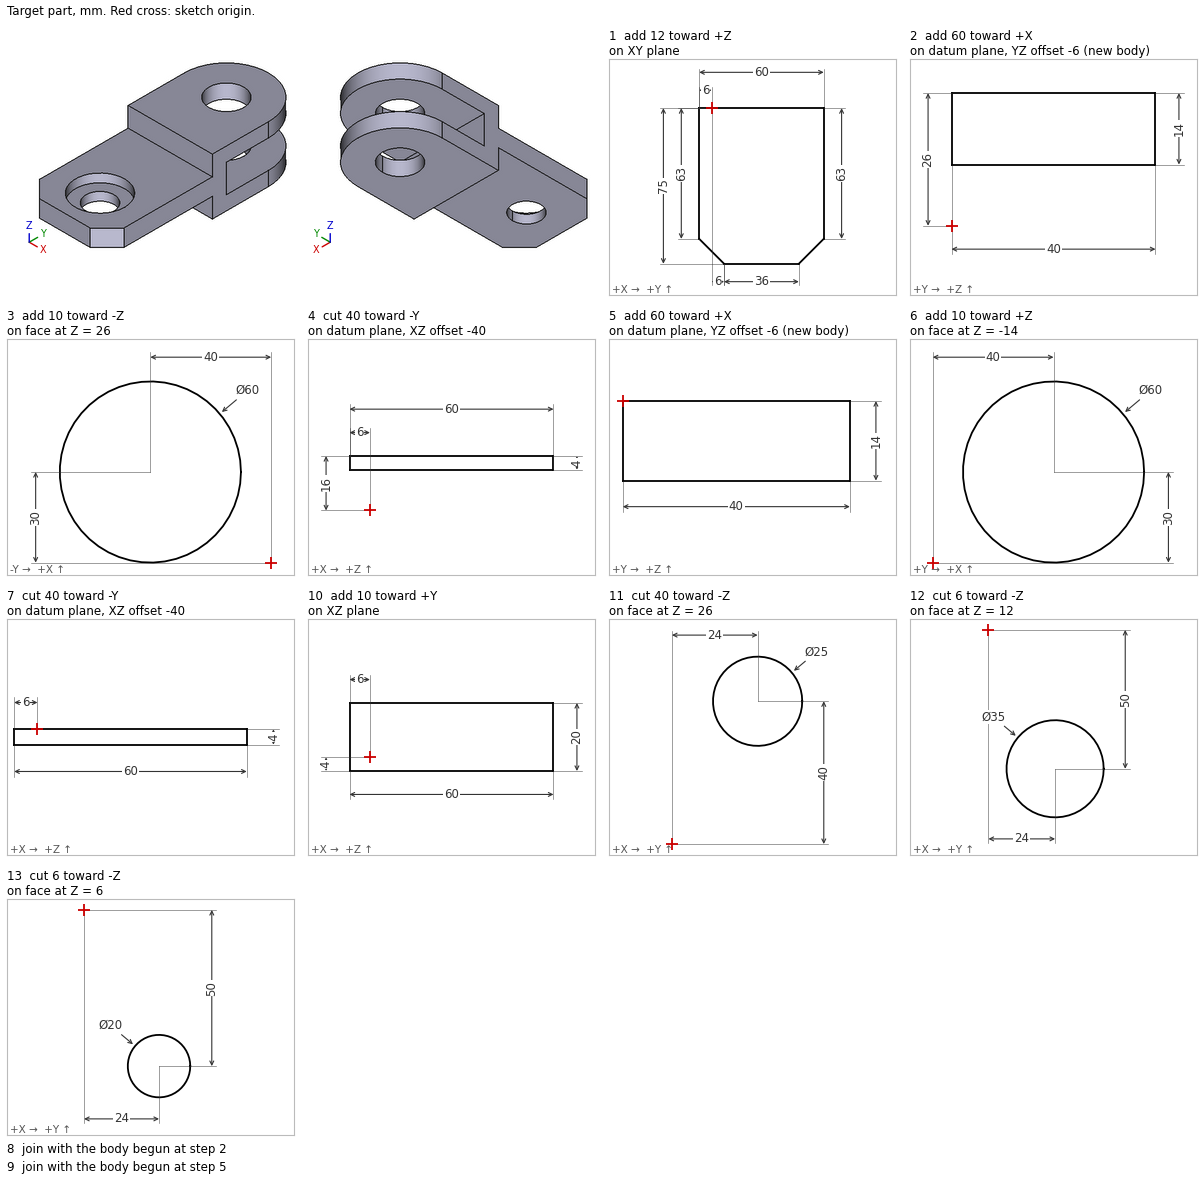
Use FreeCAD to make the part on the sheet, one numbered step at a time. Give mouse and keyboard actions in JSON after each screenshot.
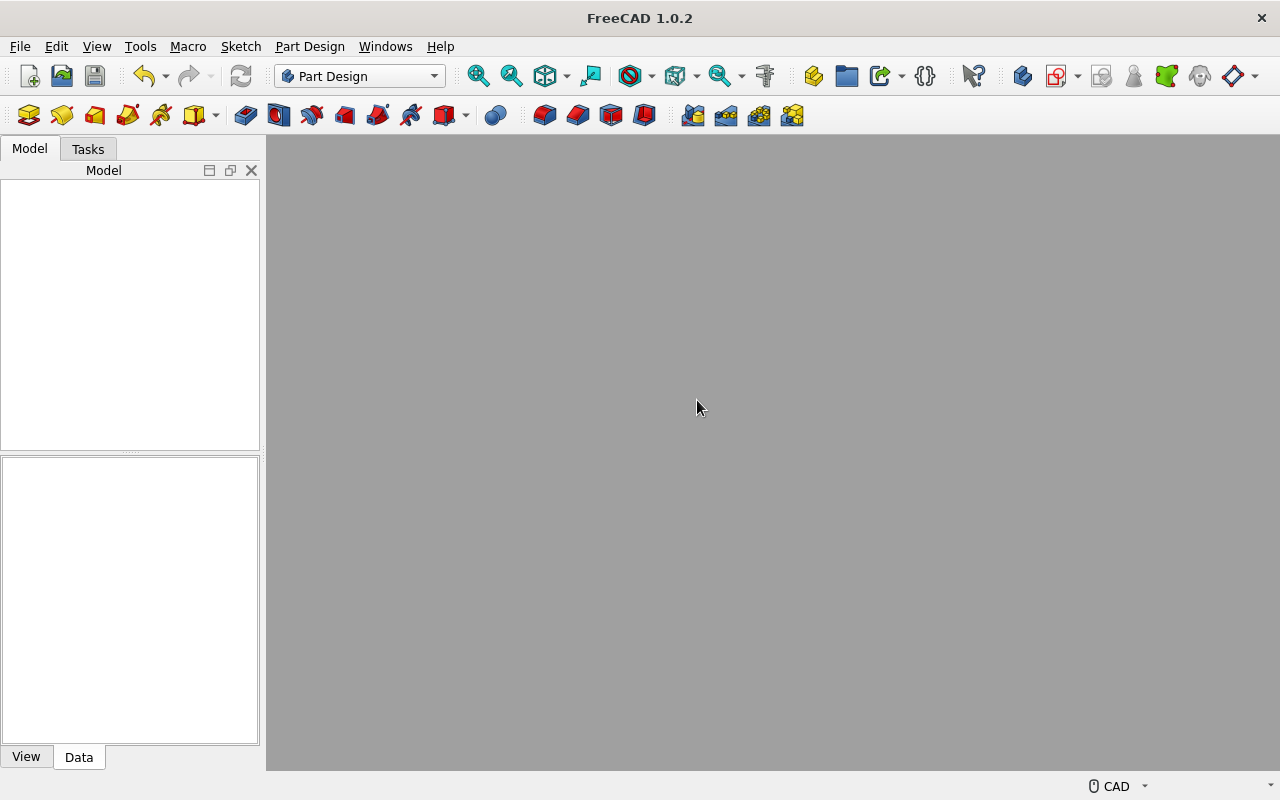
{"action": "left_click", "coordinate": [29, 76]}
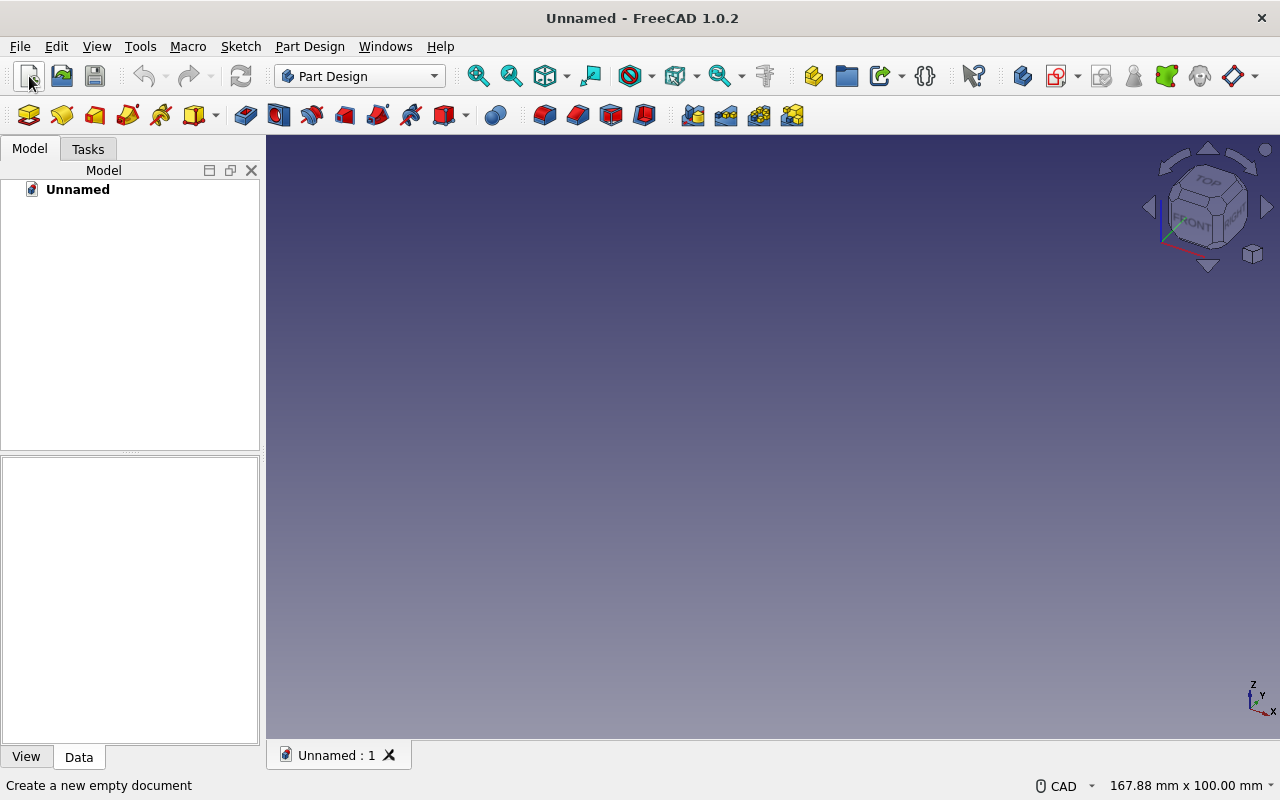
{"action": "left_click", "coordinate": [1056, 76]}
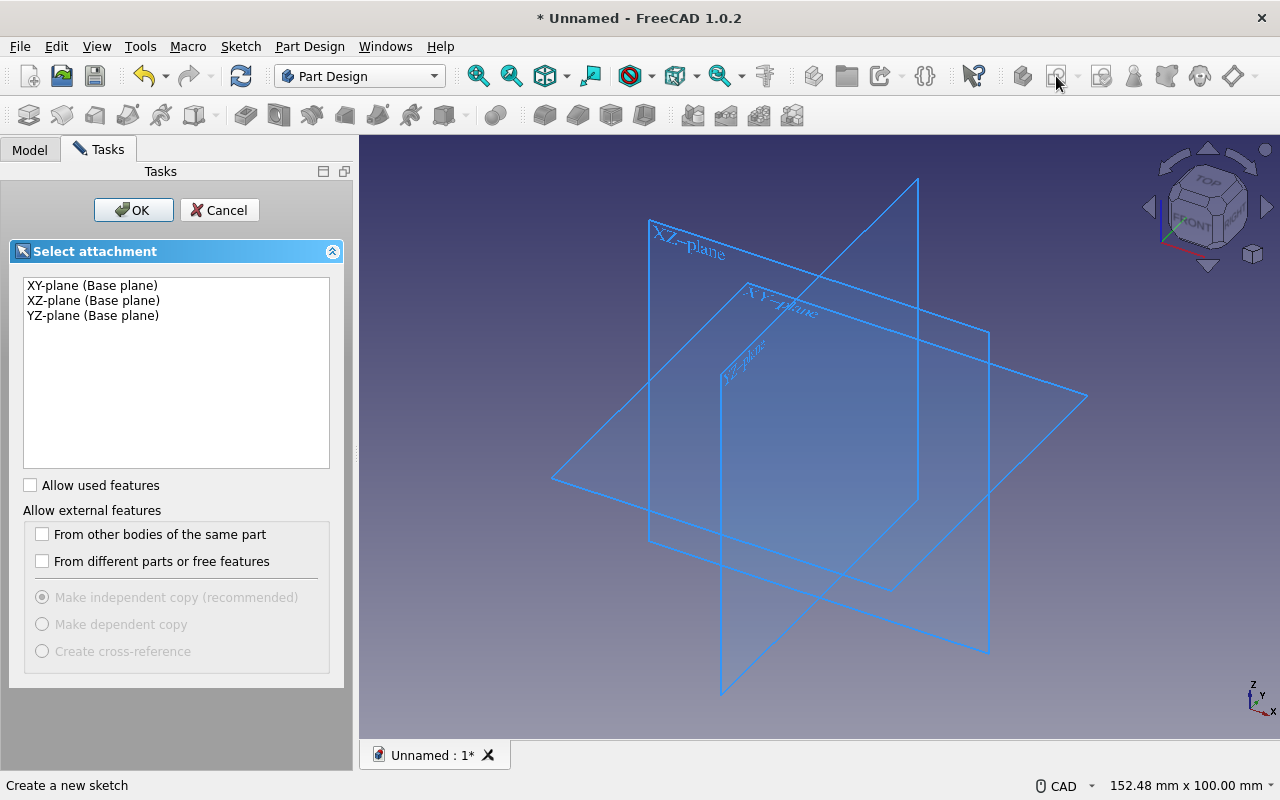
{"action": "left_click", "coordinate": [84, 286]}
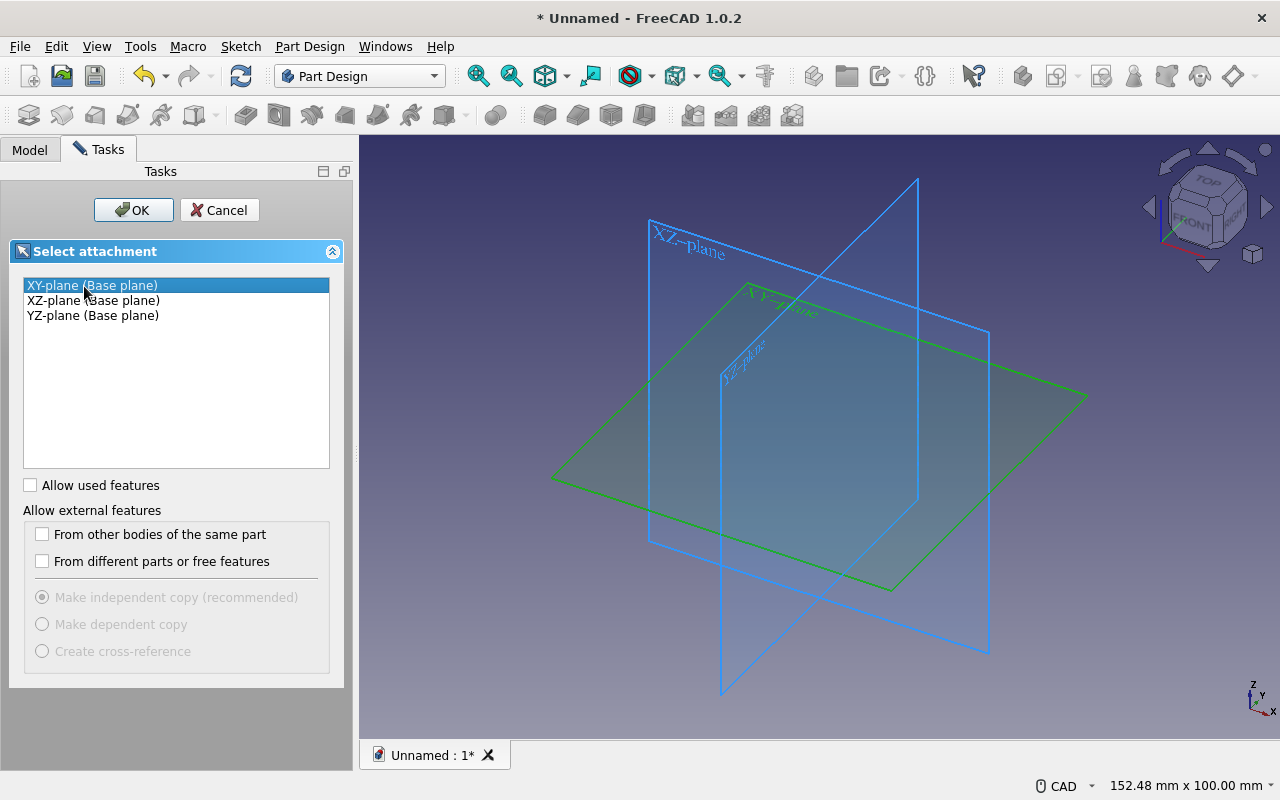
{"action": "left_click", "coordinate": [134, 210]}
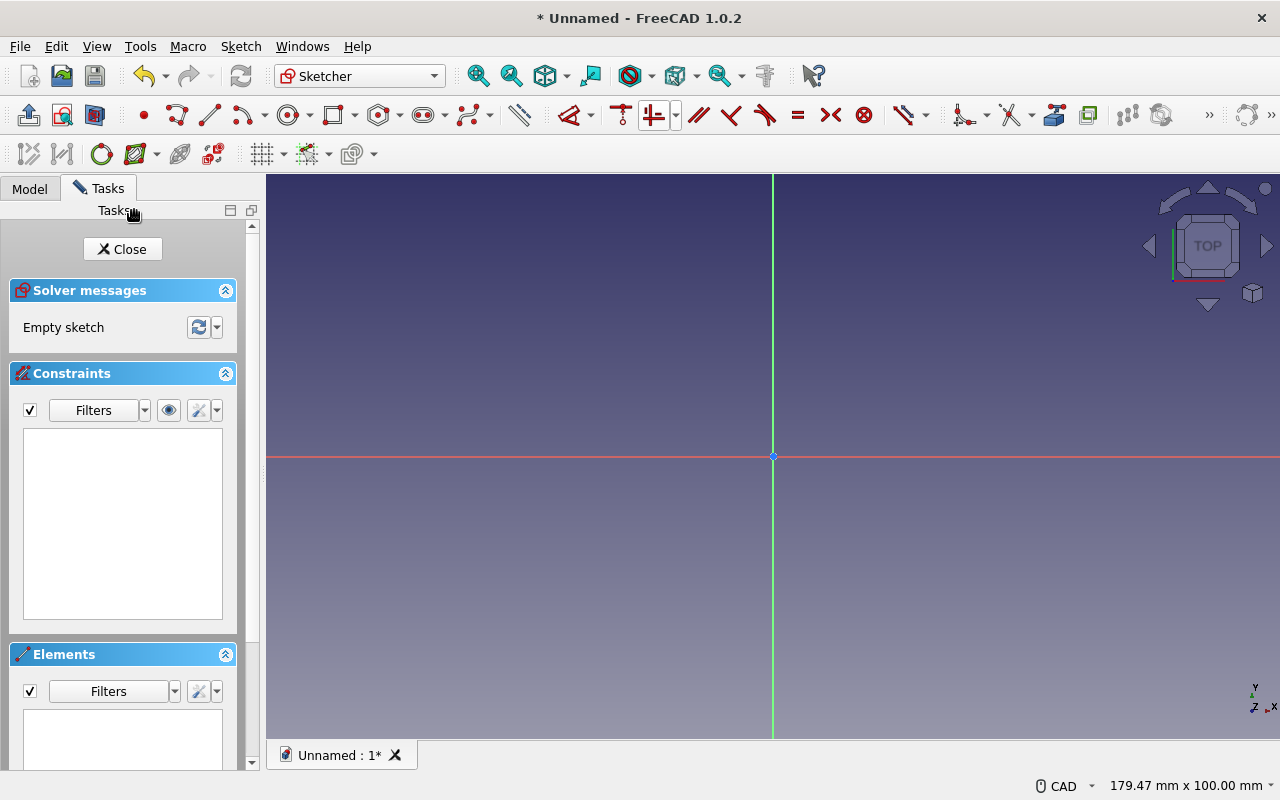
{"action": "scroll", "coordinate": [294, 202], "scroll_direction": "down", "scroll_amount": 2}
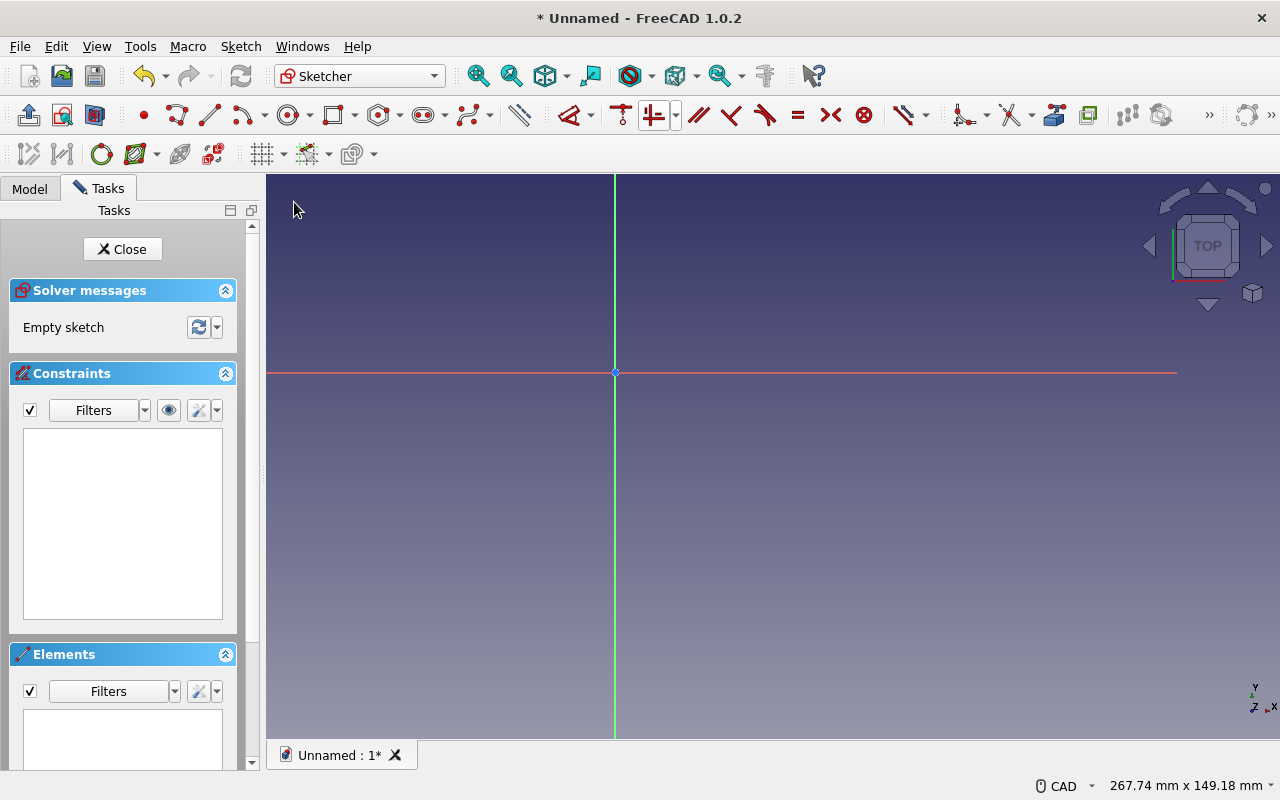
{"action": "left_click", "coordinate": [177, 116]}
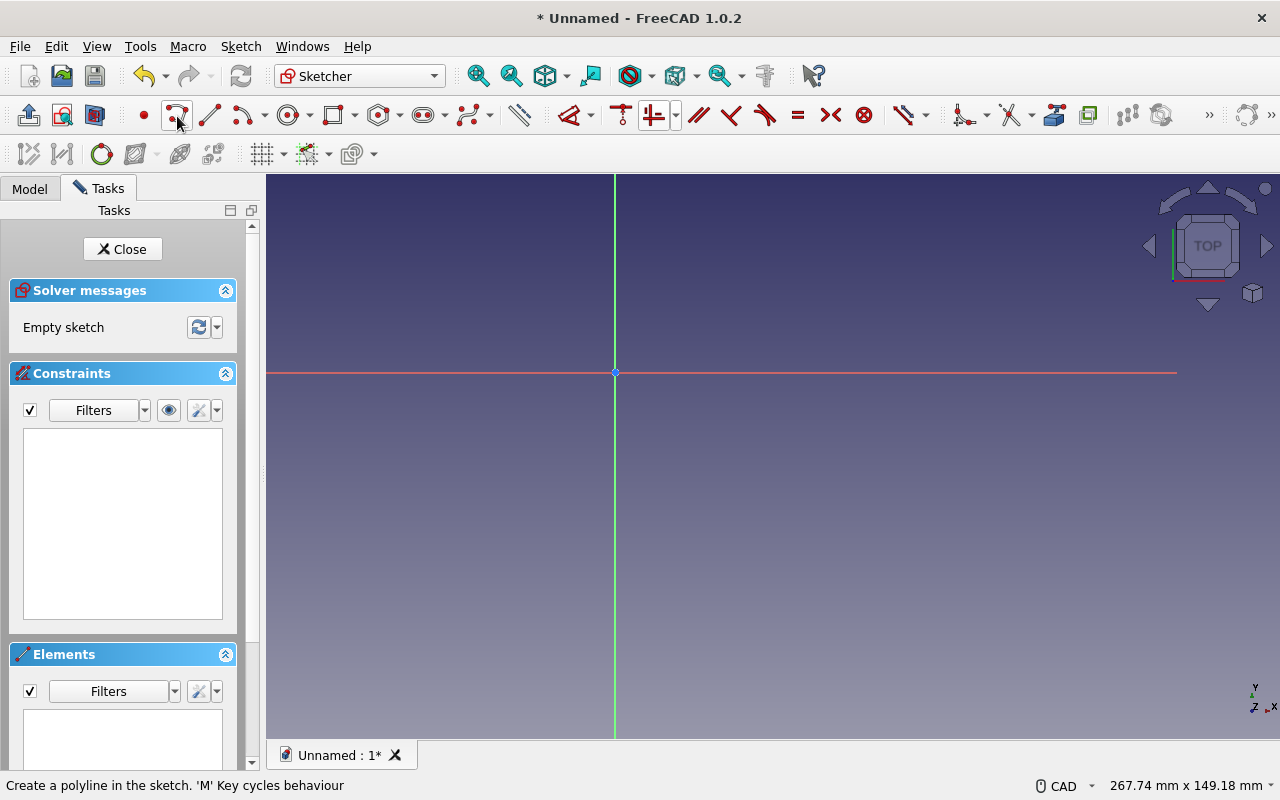
{"action": "left_click", "coordinate": [592, 373]}
{"action": "left_click", "coordinate": [592, 611]}
{"action": "left_click", "coordinate": [638, 657]}
{"action": "left_click", "coordinate": [774, 657]}
{"action": "left_click", "coordinate": [820, 611]}
{"action": "left_click", "coordinate": [820, 382]}
{"action": "left_click", "coordinate": [592, 373]}
{"action": "key", "text": "Escape"}
{"action": "key", "text": "Escape"}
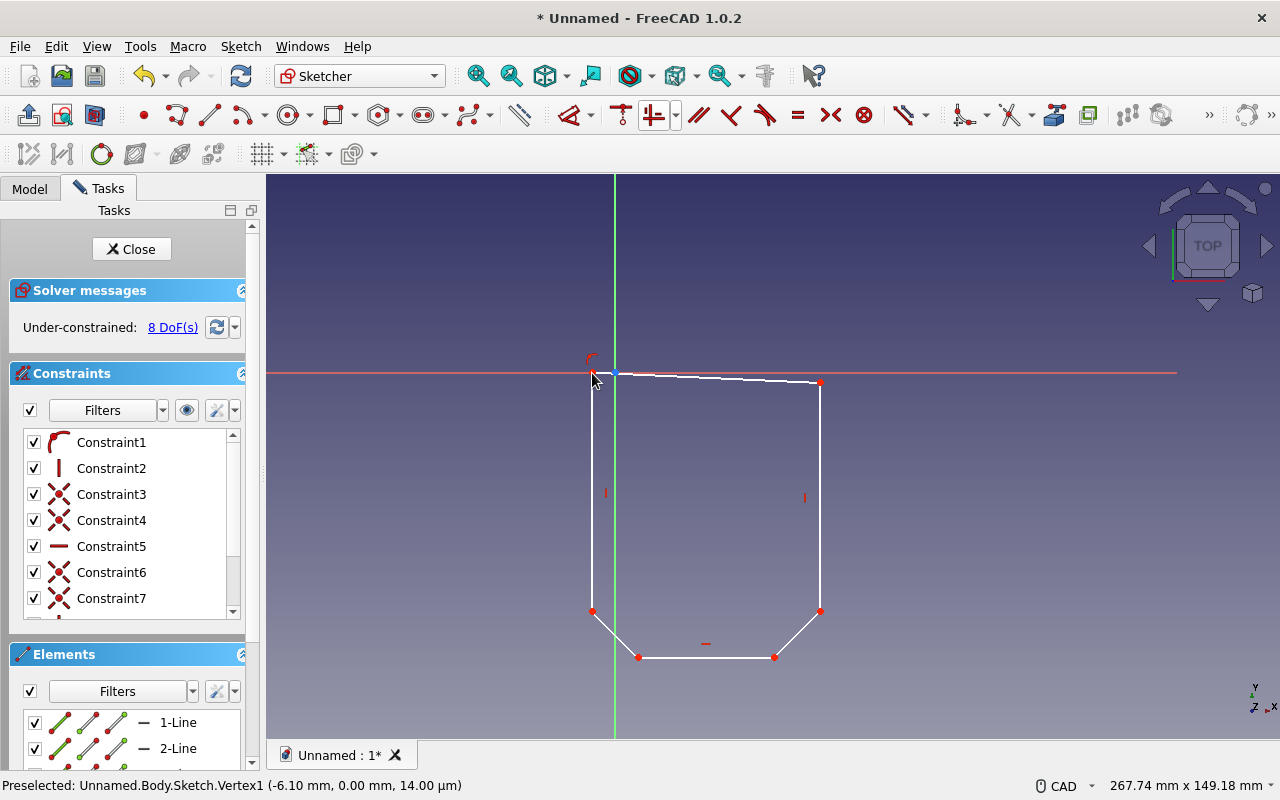
{"action": "left_click", "coordinate": [660, 376]}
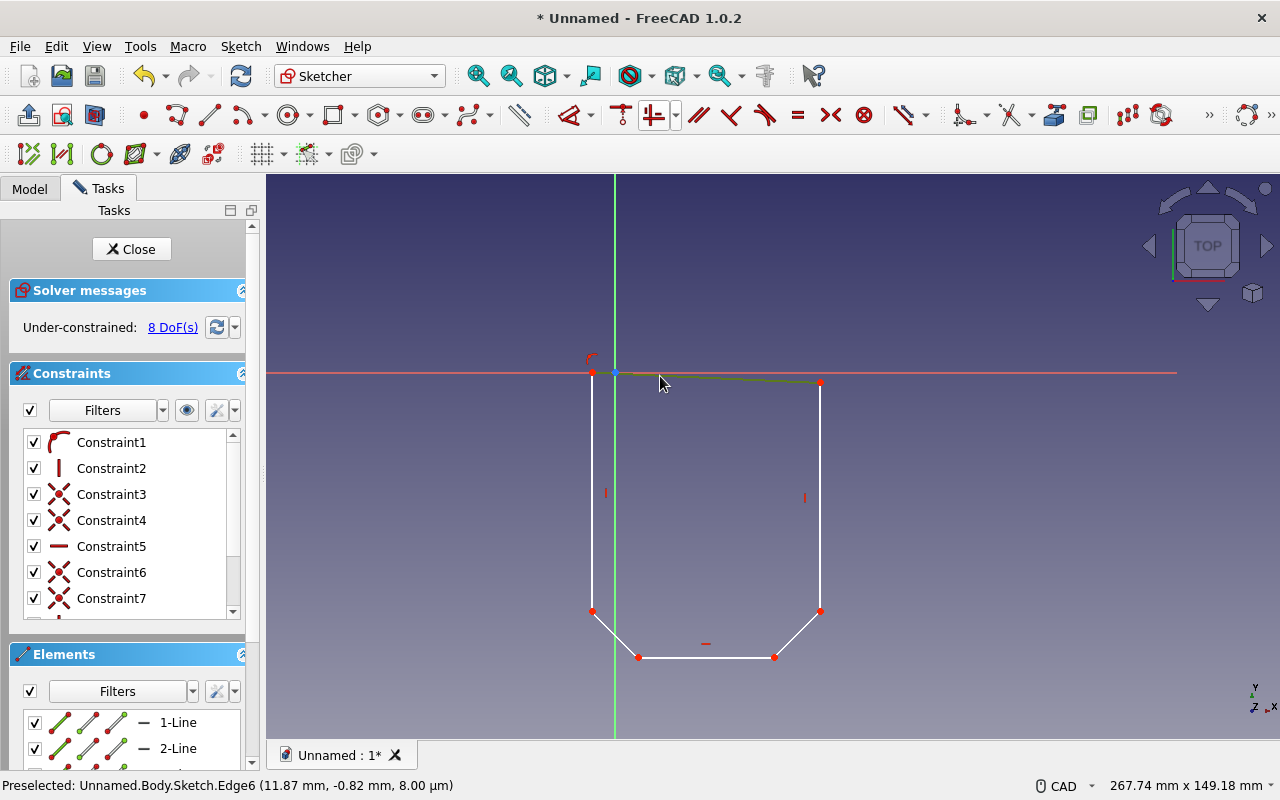
{"action": "key", "text": "h"}